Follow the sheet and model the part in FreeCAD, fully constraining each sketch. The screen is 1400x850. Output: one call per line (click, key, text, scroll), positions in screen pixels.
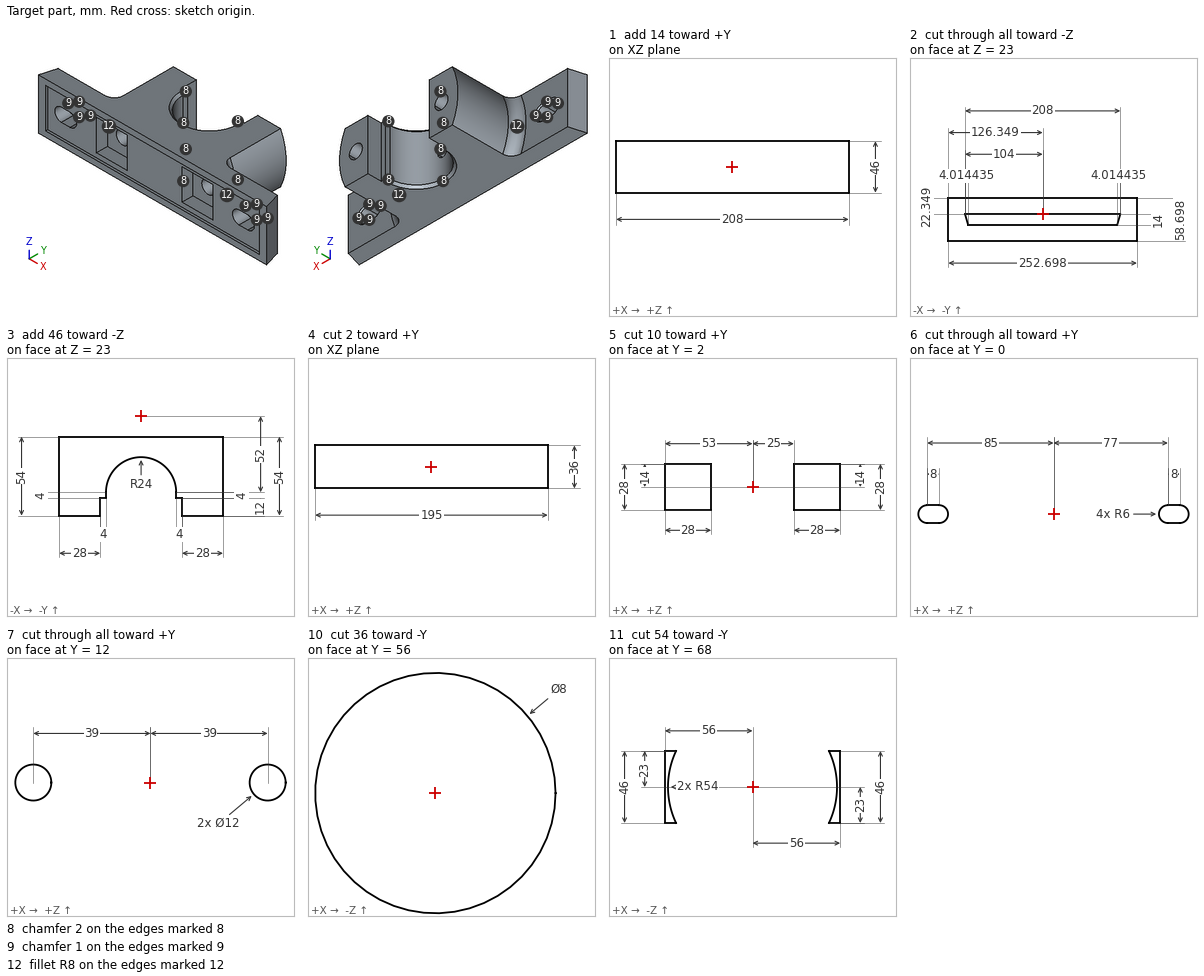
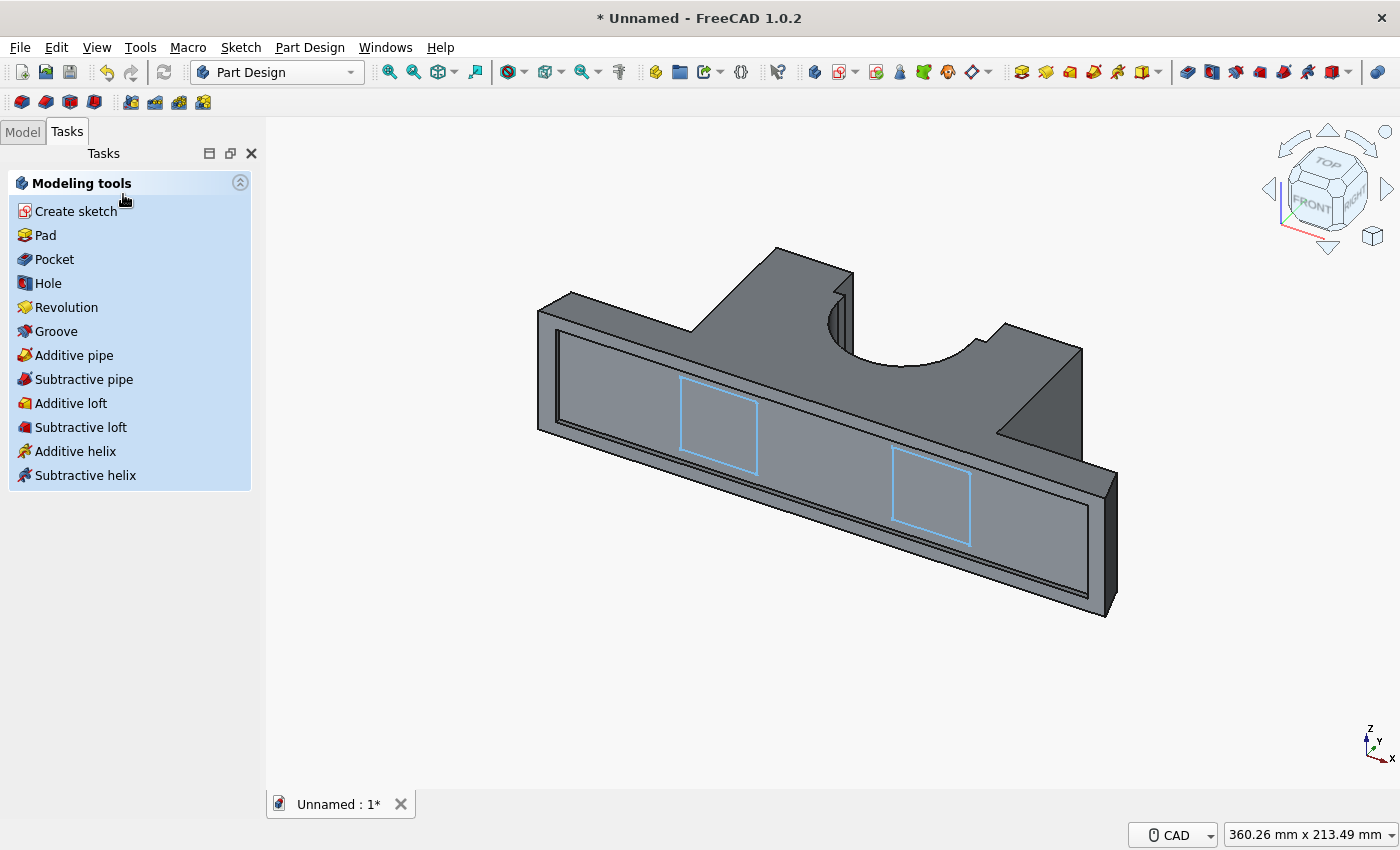
click(1188, 72)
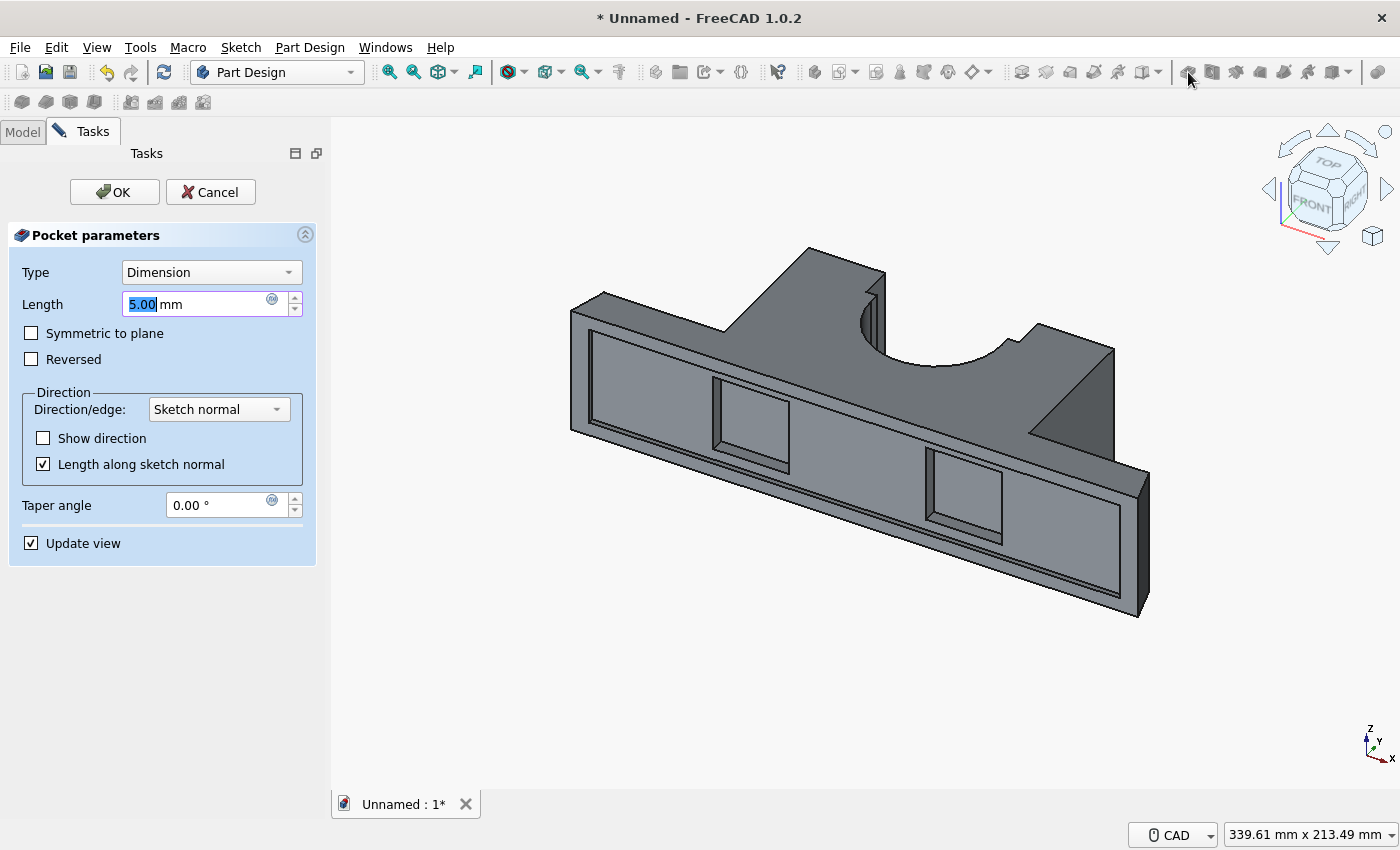
text(10)
key(Tab)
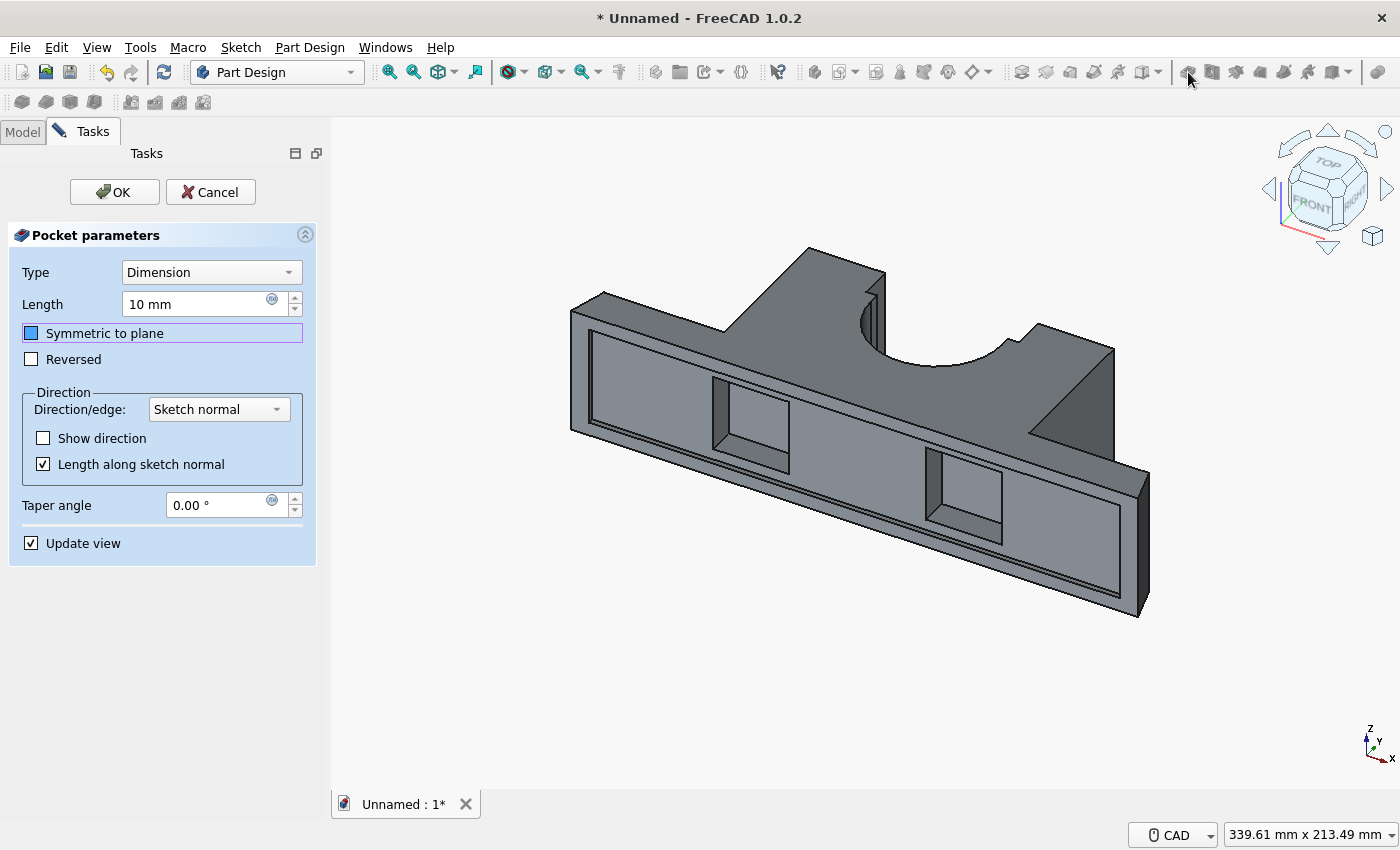
click(115, 192)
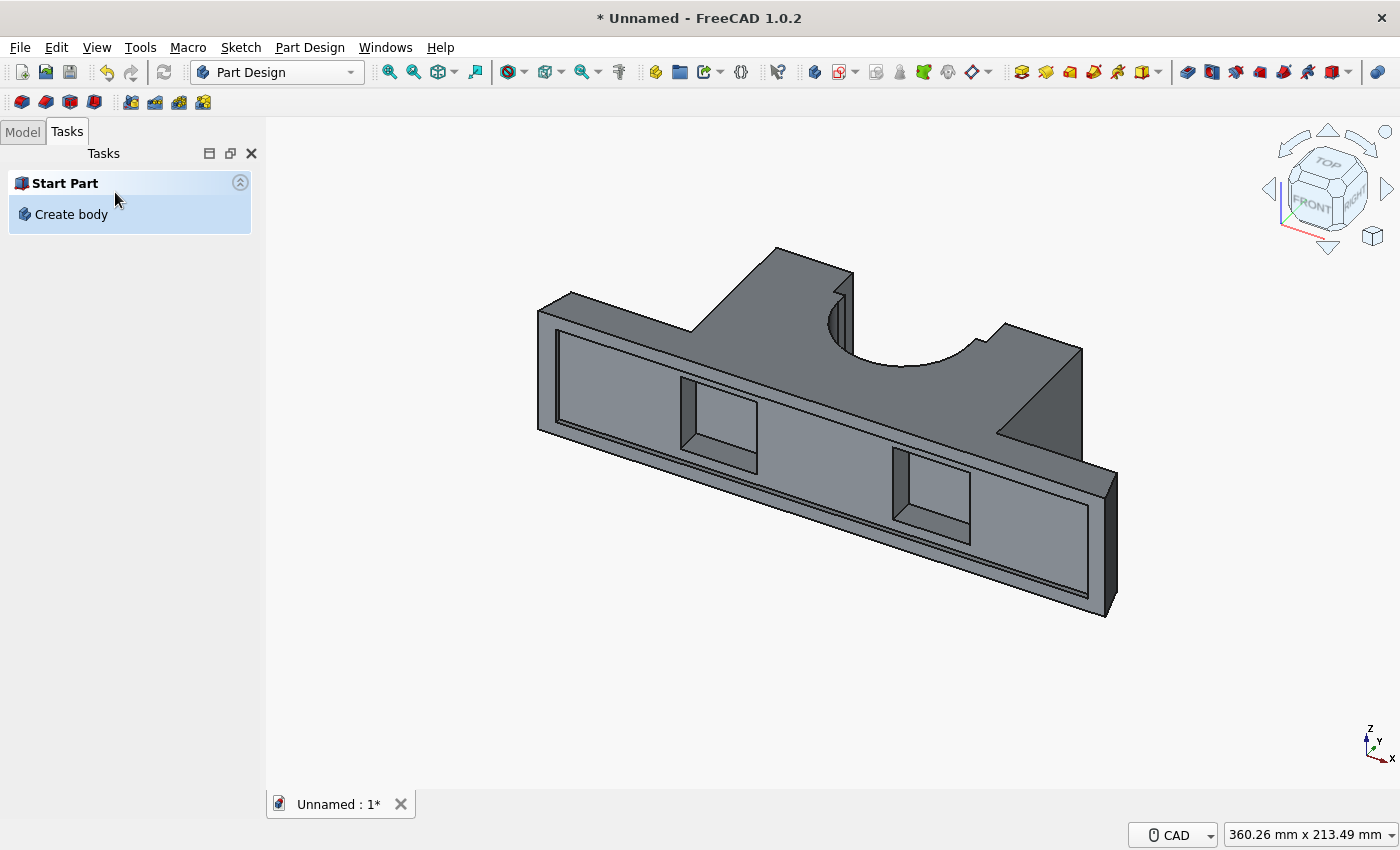
scroll(1065, 493, up, 4)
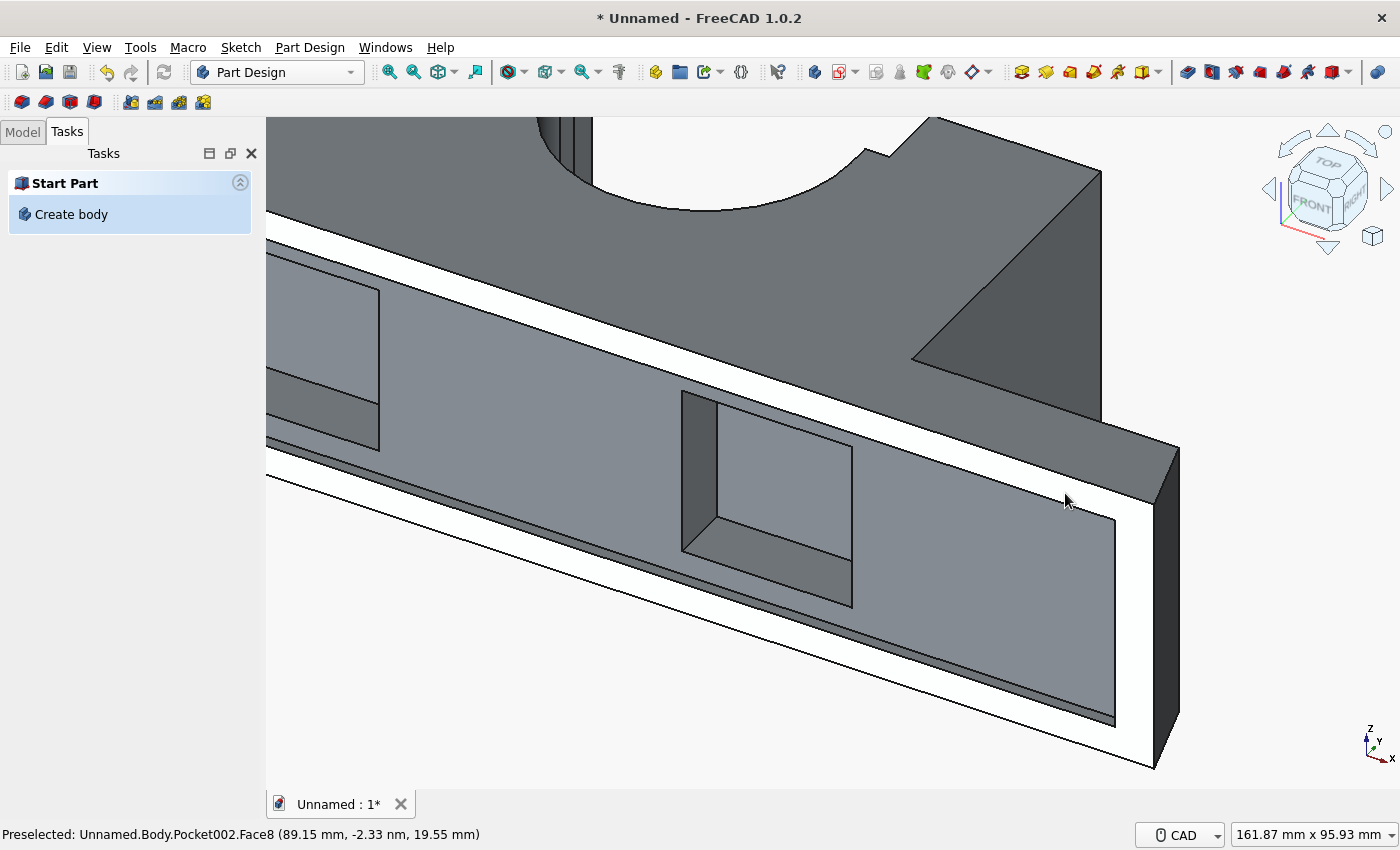
click(1064, 493)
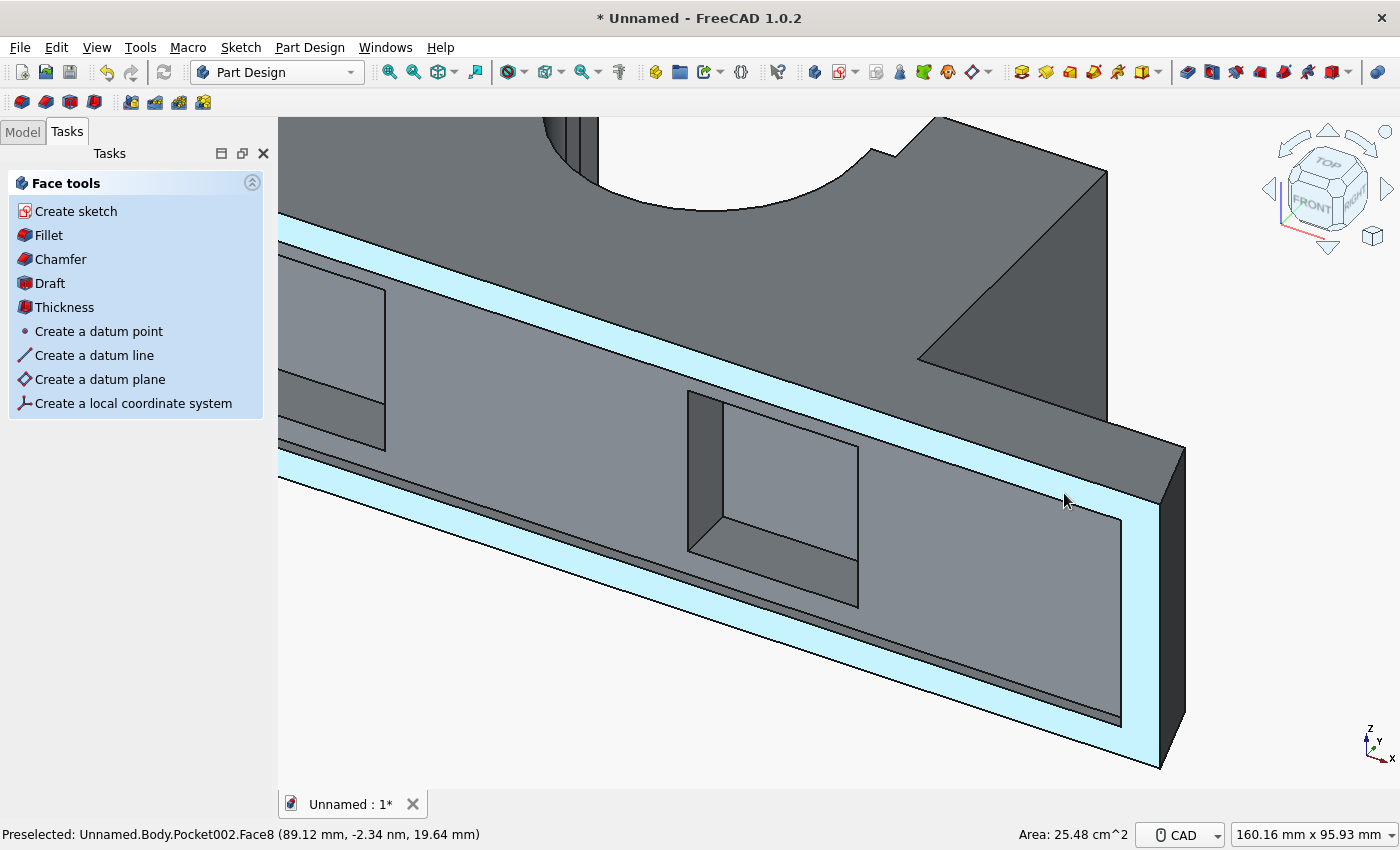
click(840, 72)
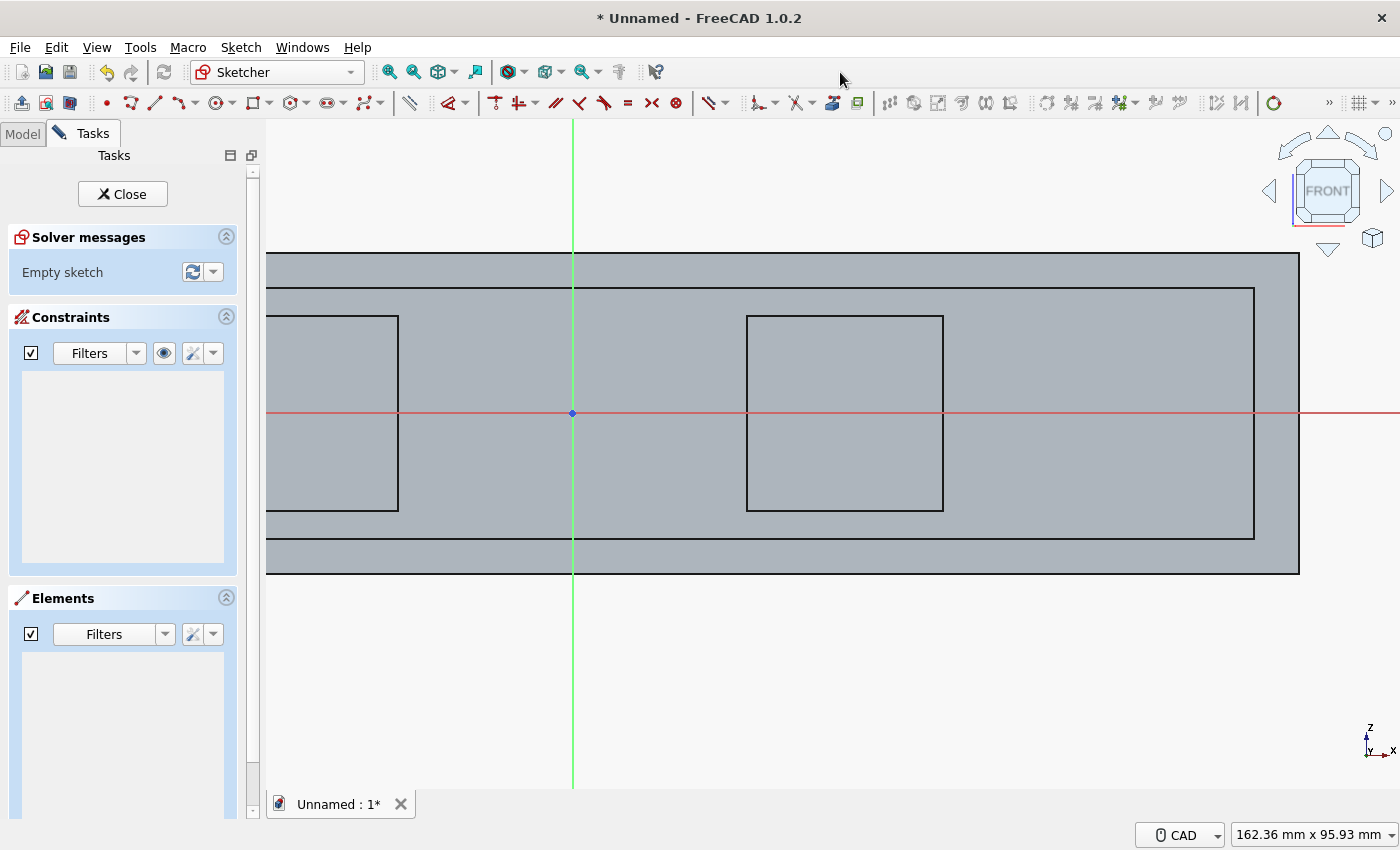
scroll(998, 503, down, 3)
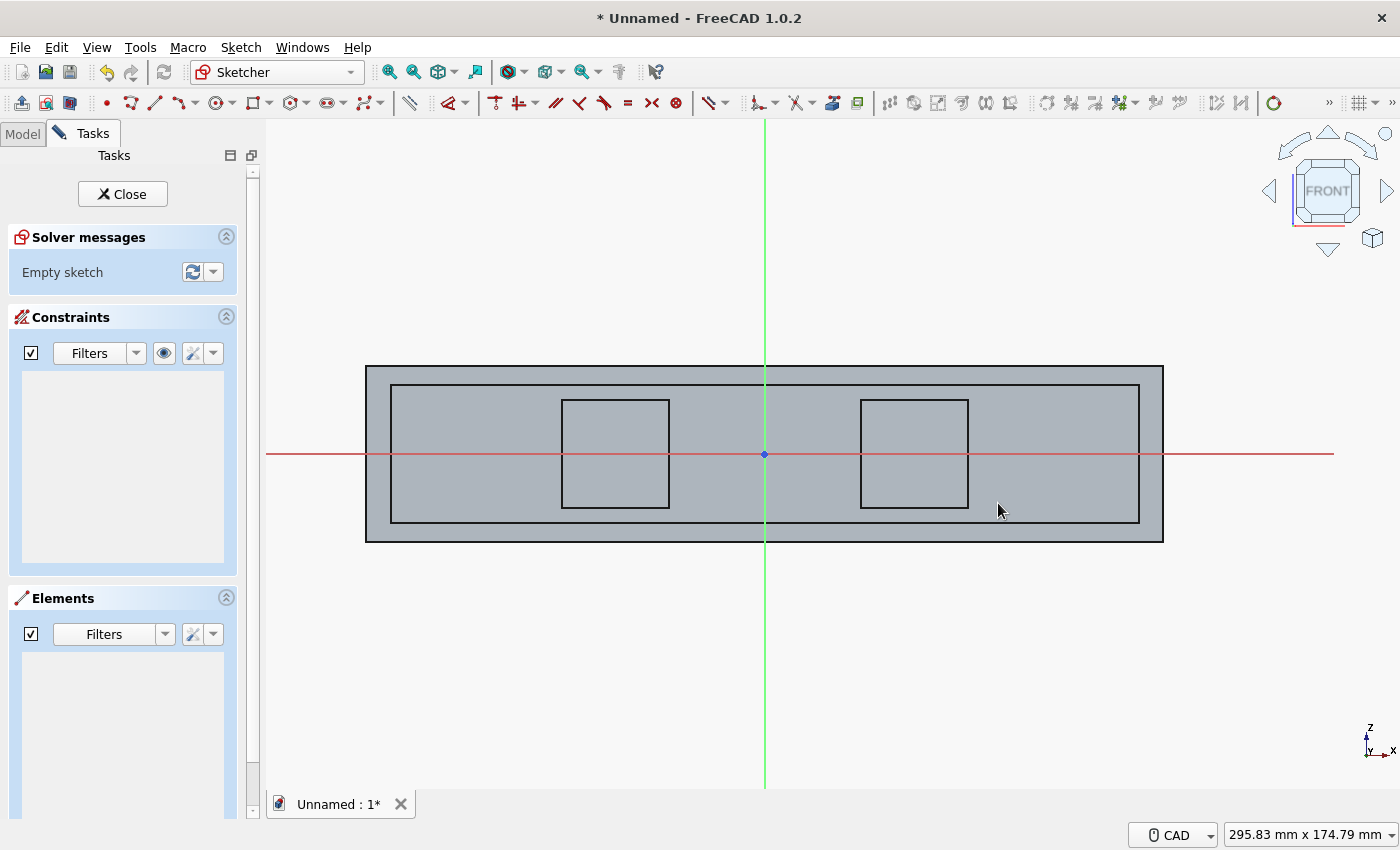
key(g)
key(s)